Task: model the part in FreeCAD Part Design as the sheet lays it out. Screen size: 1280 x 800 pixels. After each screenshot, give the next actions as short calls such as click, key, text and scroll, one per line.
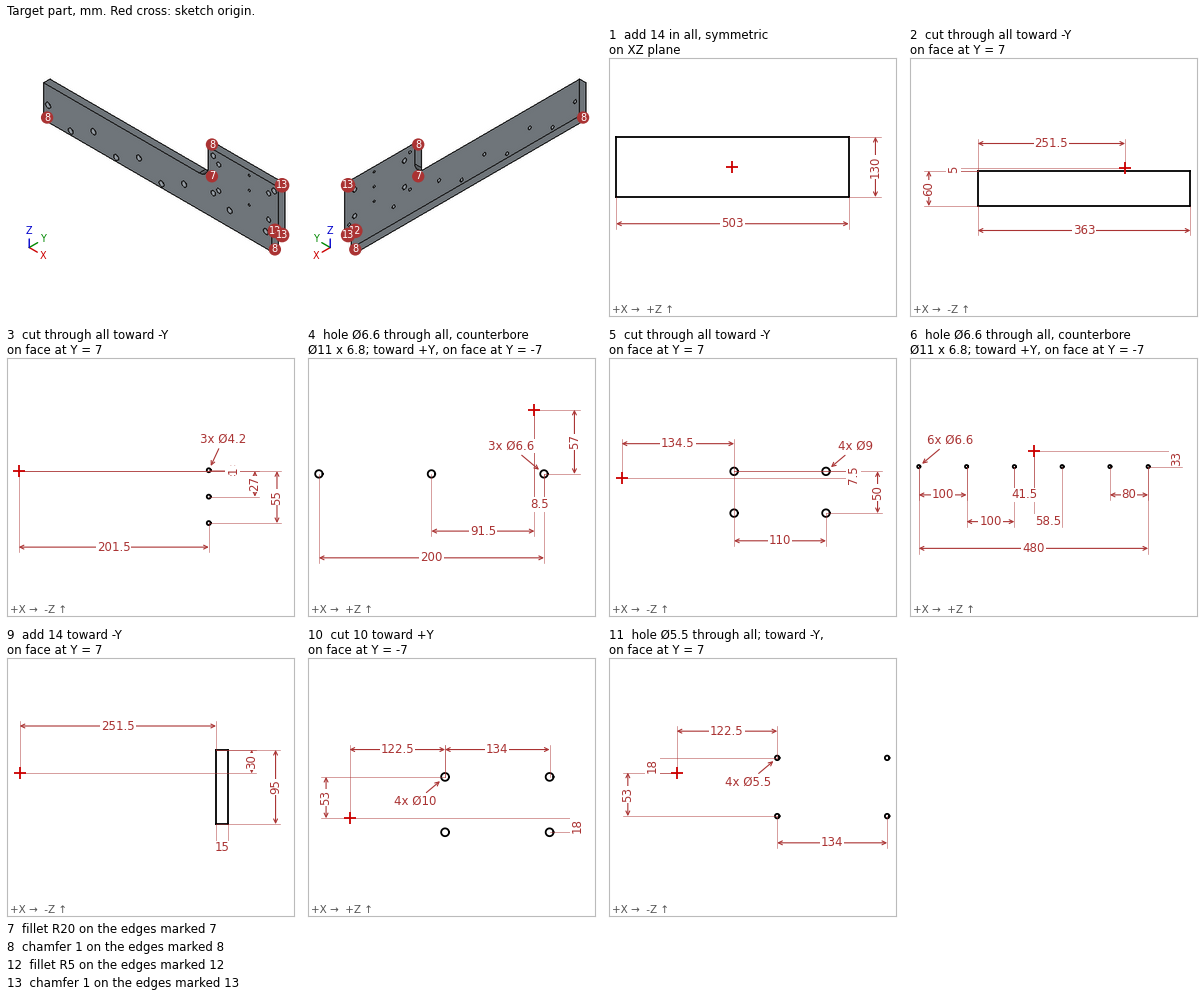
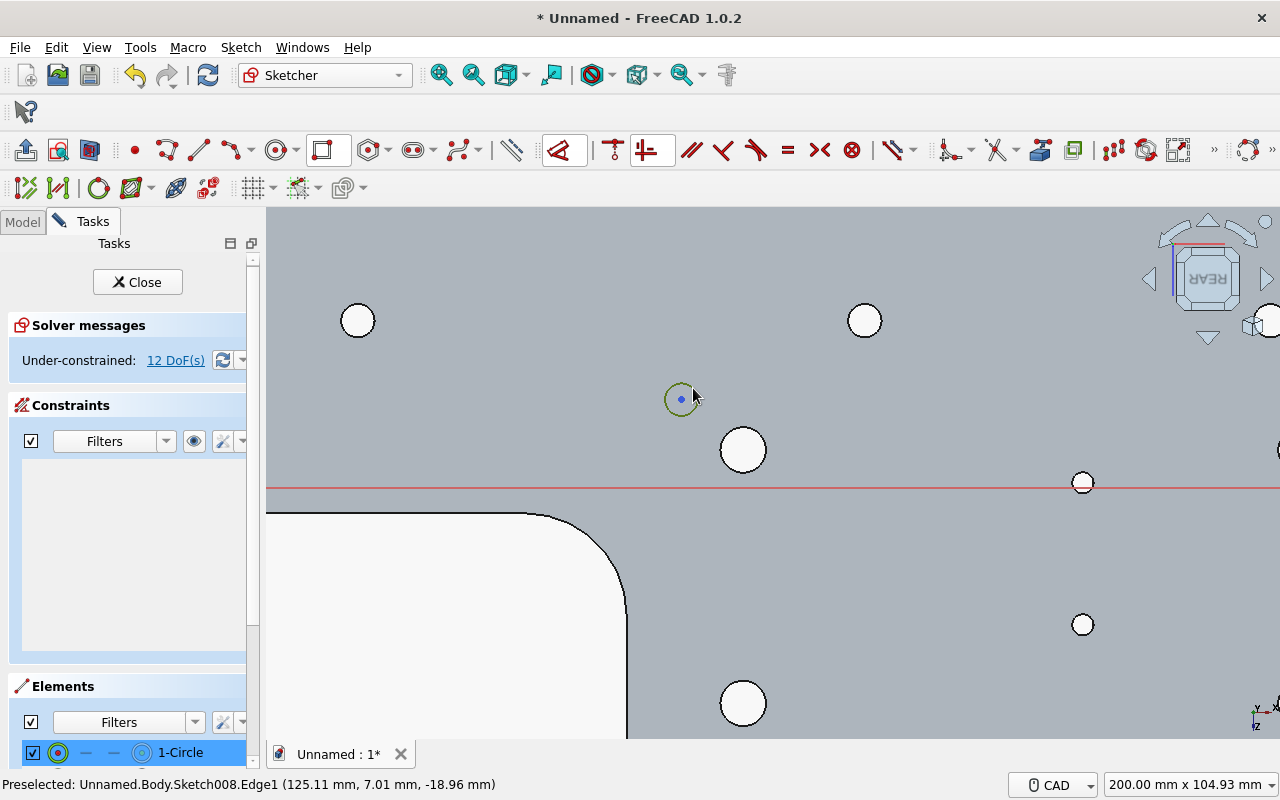
scroll(693, 388, down, 4)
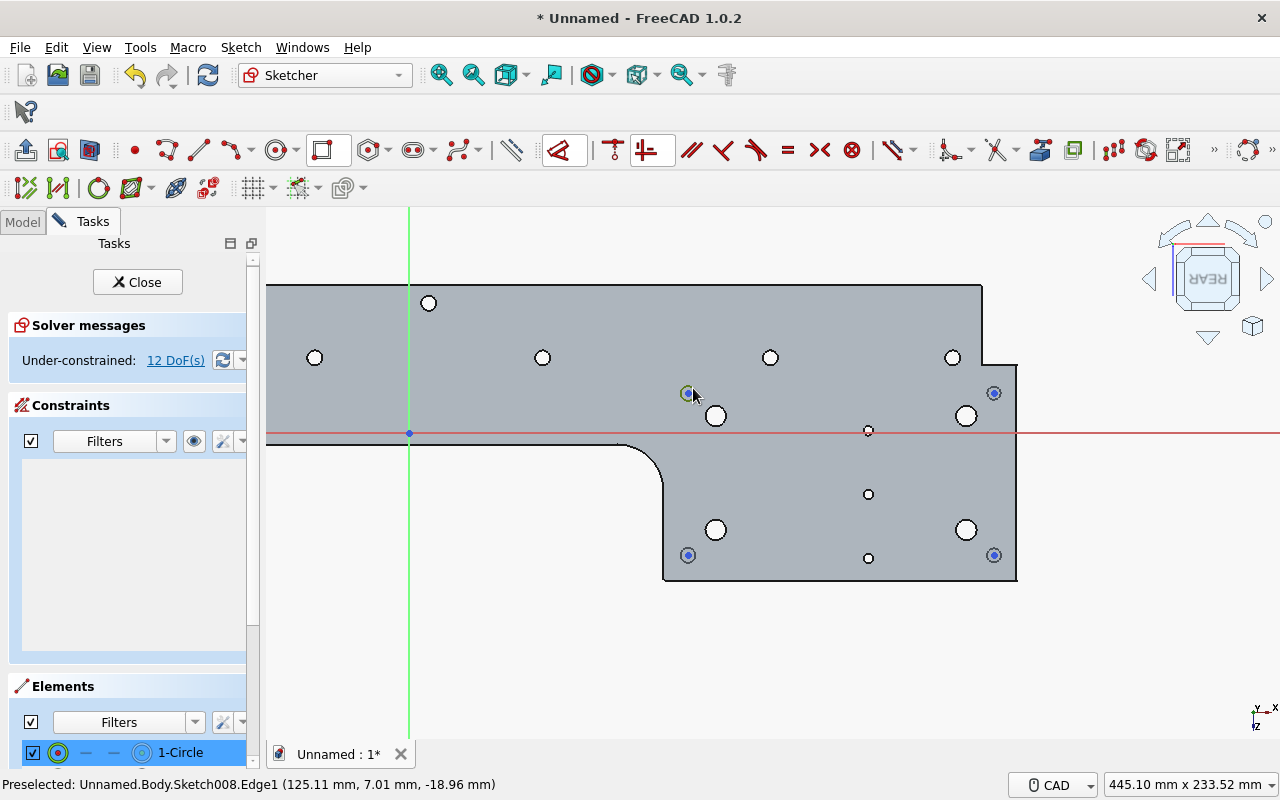
scroll(693, 550, up, 4)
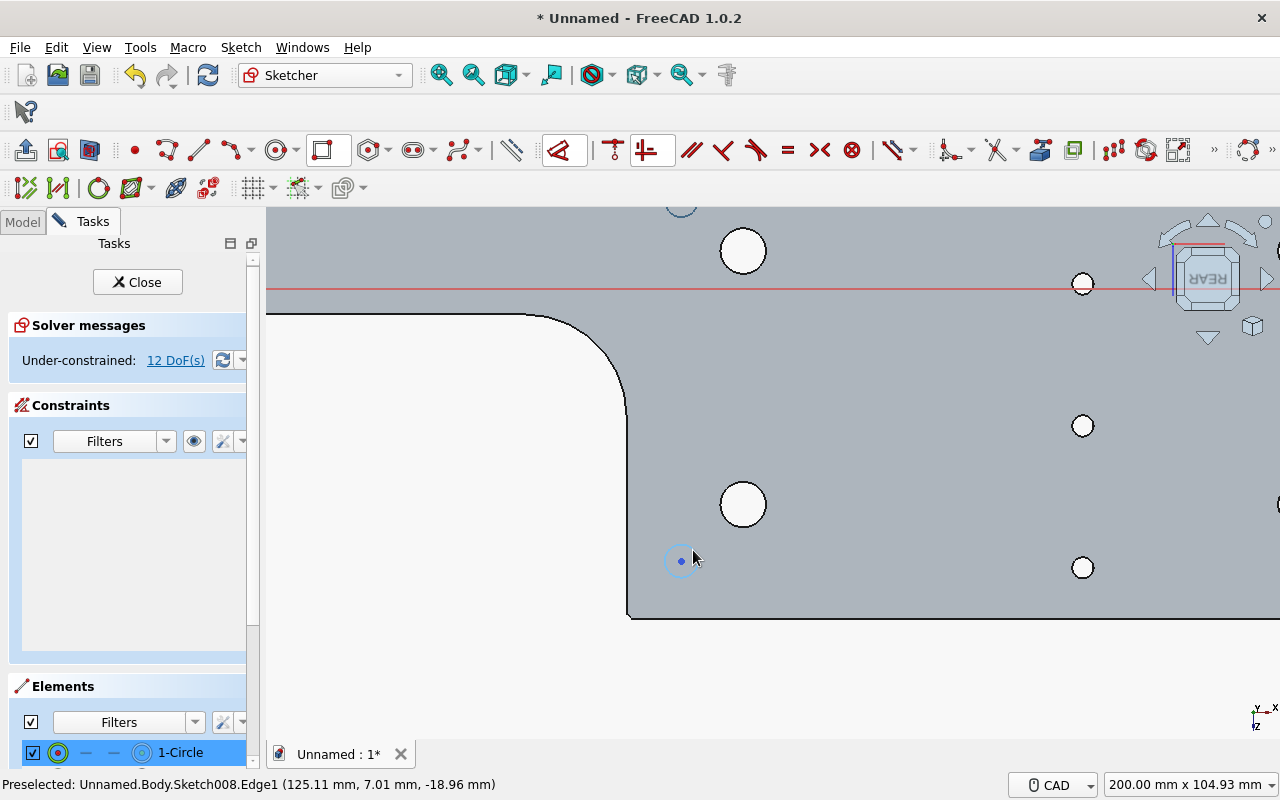
click(693, 549)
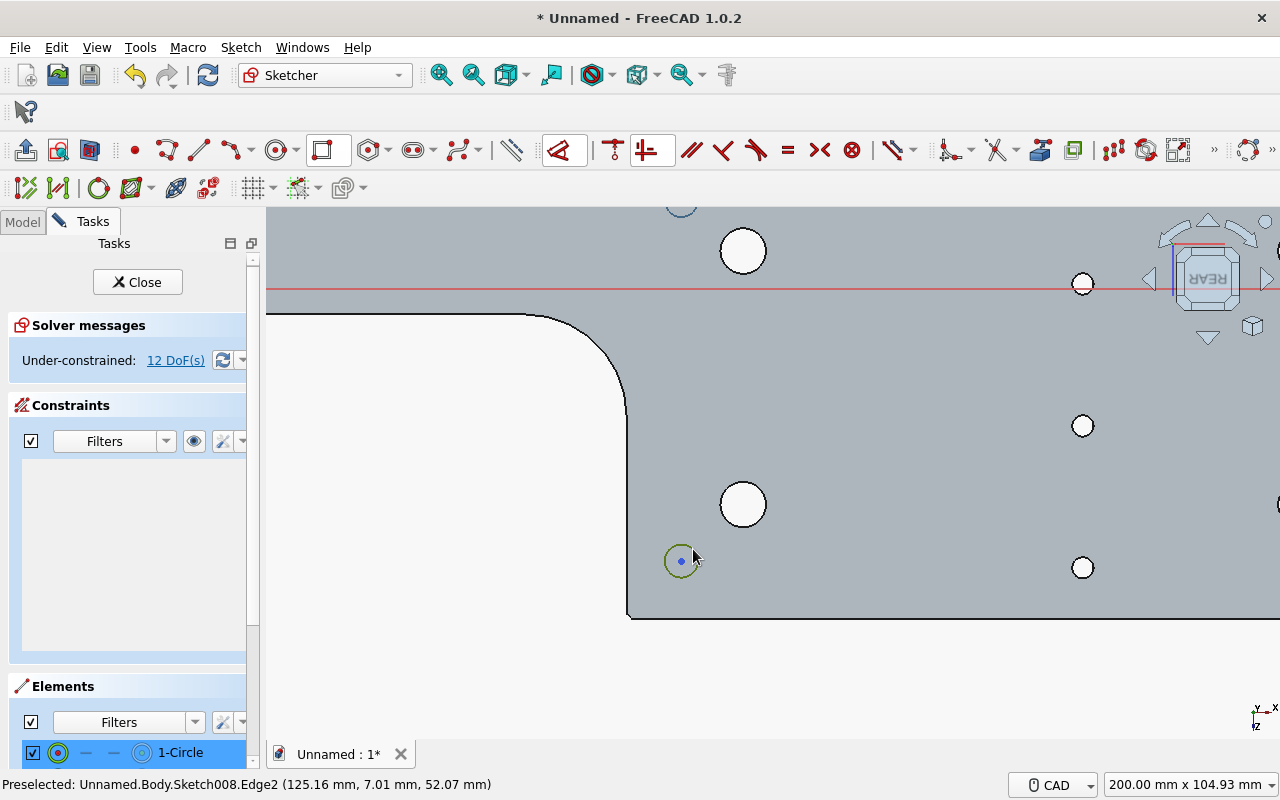
scroll(693, 551, down, 4)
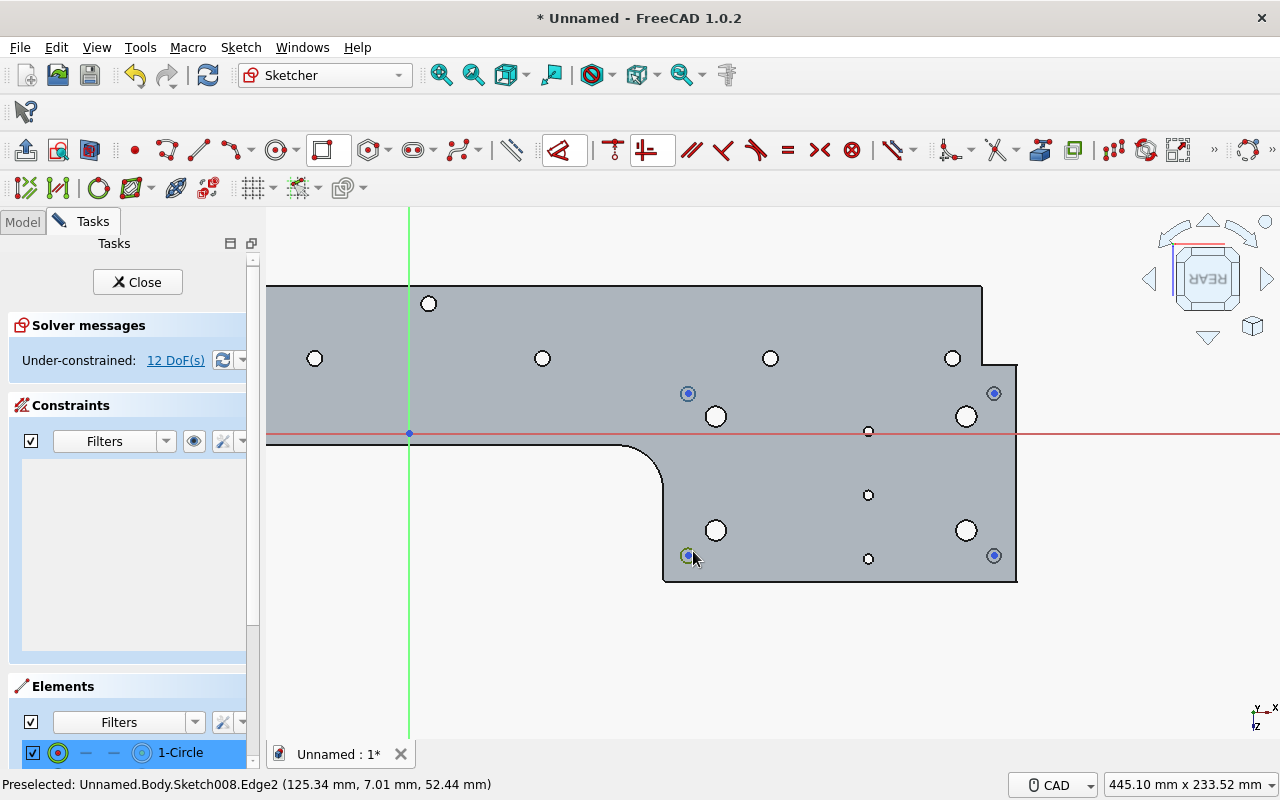
scroll(999, 551, up, 4)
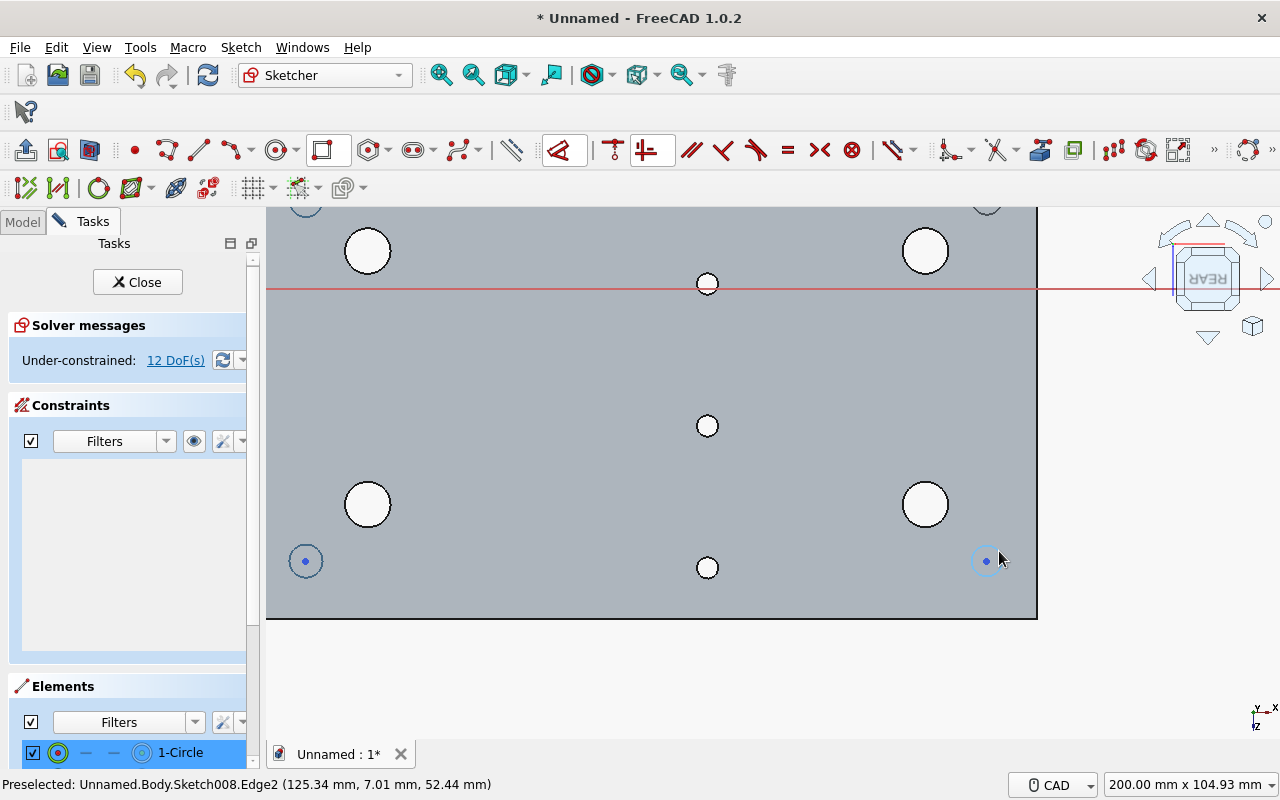
click(998, 550)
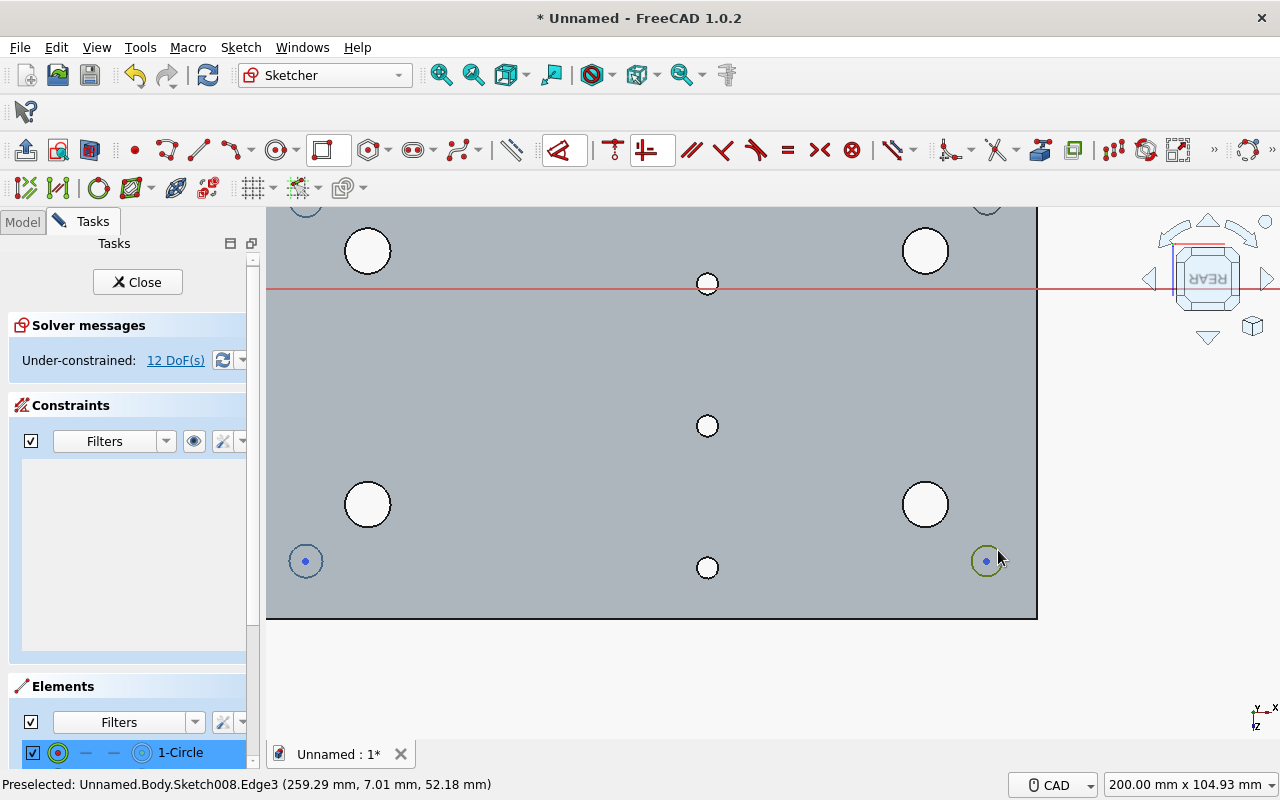
scroll(999, 551, down, 4)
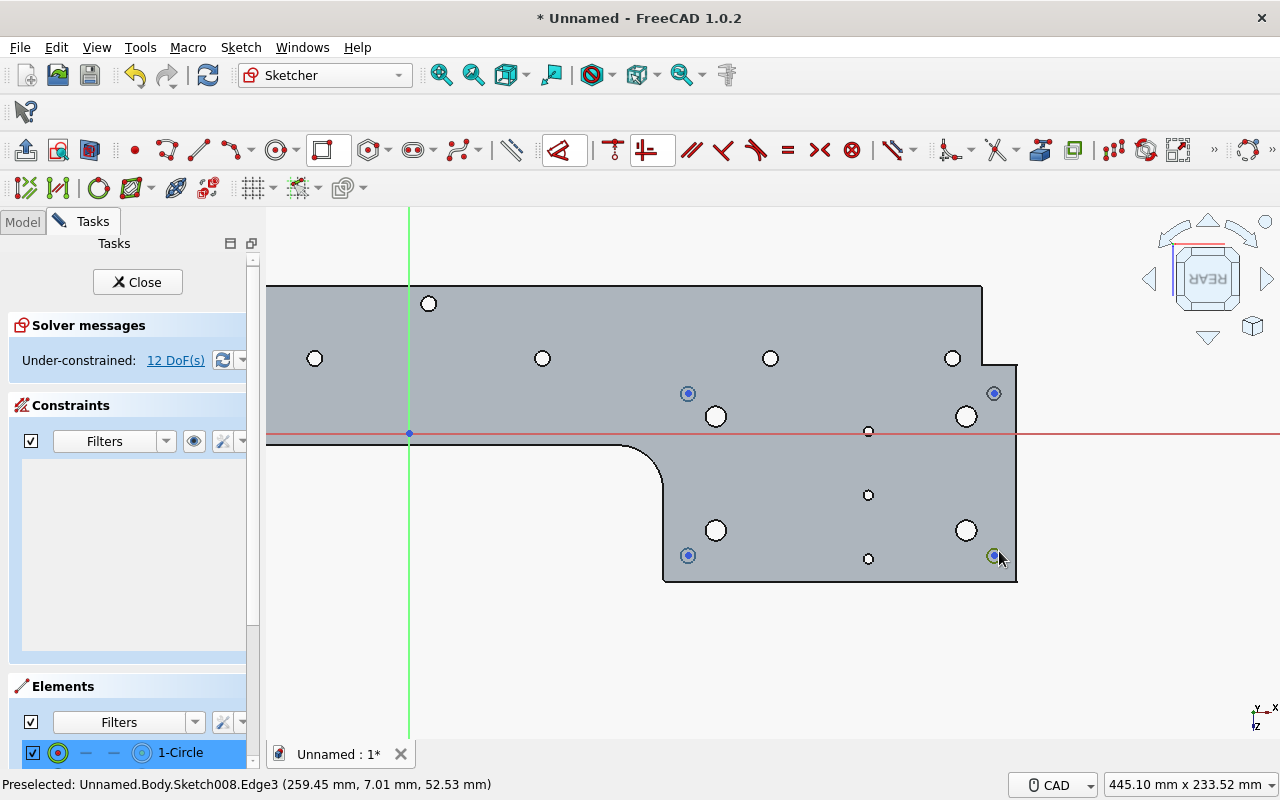
scroll(999, 389, up, 4)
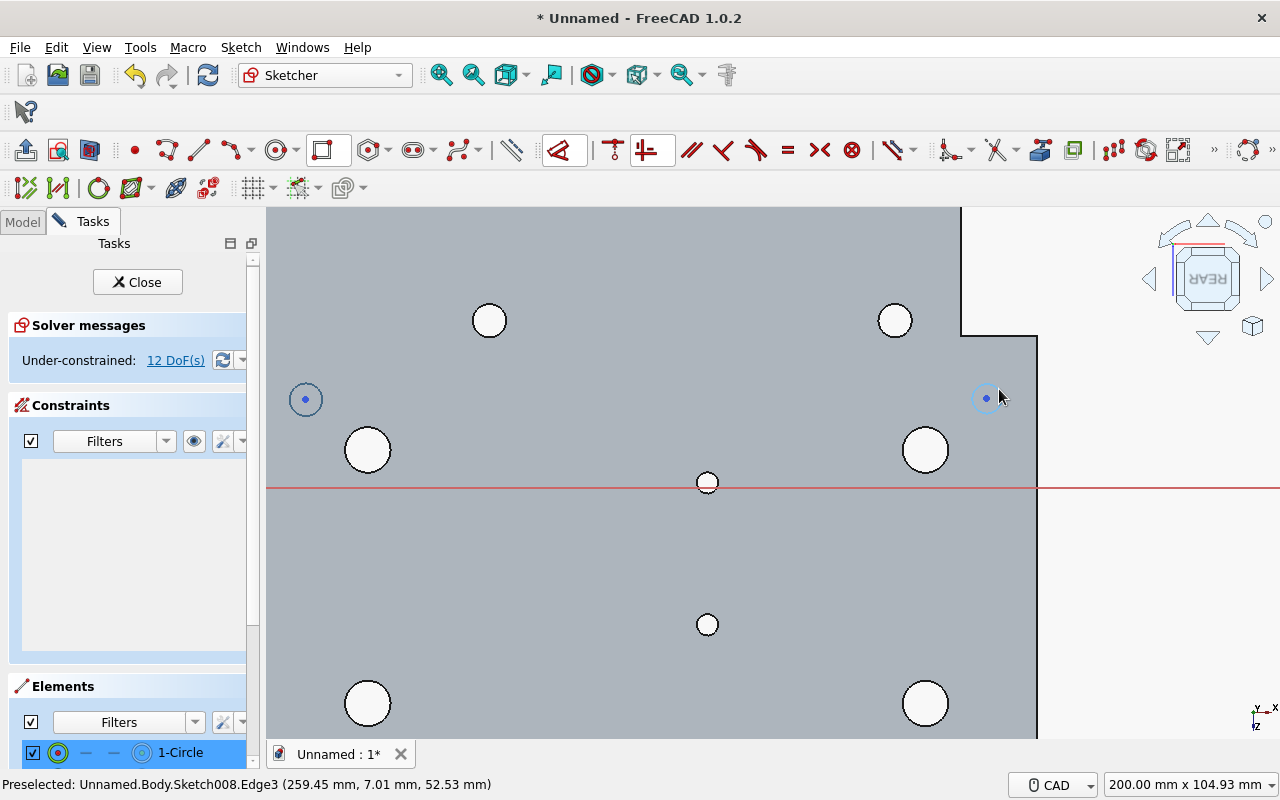
click(997, 389)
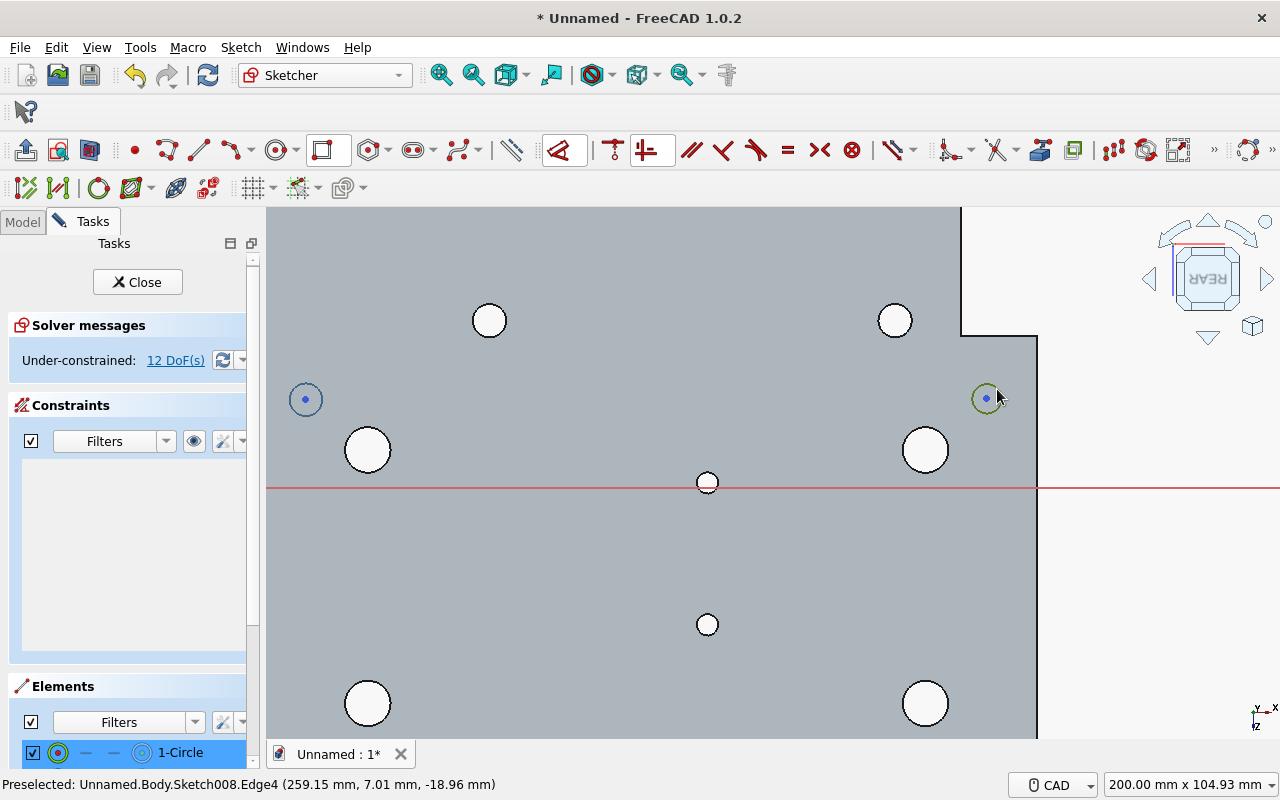
key(e)